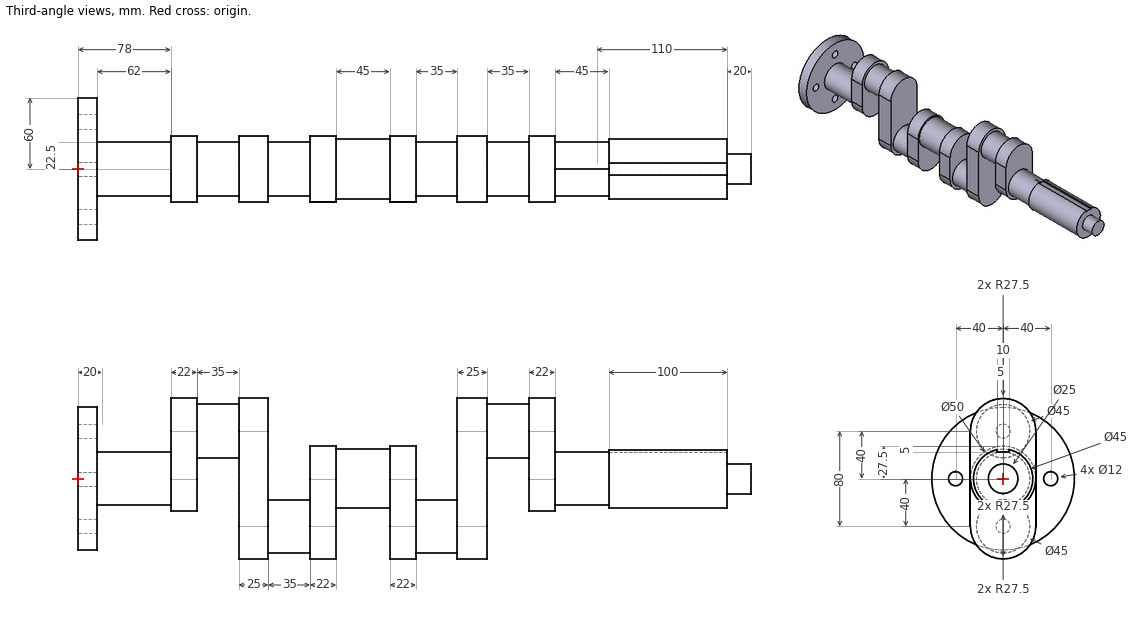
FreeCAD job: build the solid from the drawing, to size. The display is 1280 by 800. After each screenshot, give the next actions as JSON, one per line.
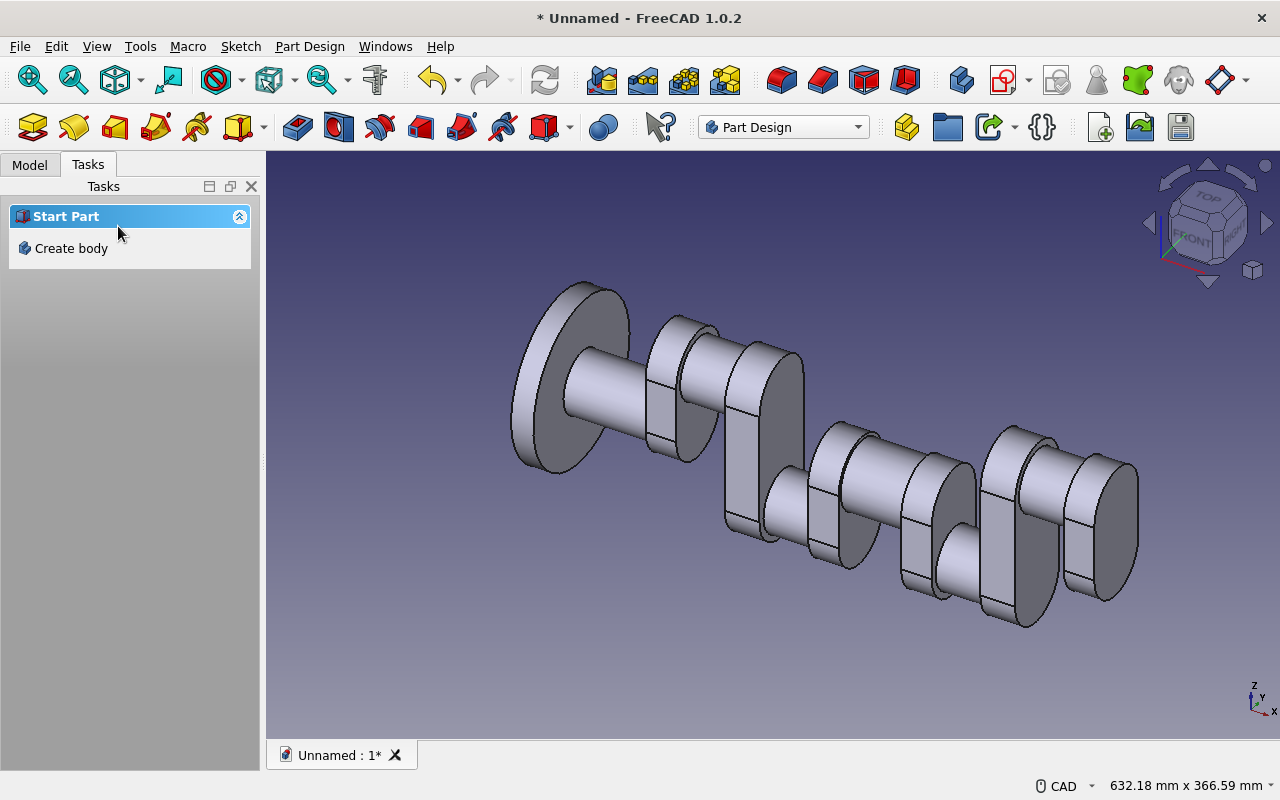
{"action": "left_click", "coordinate": [30, 164]}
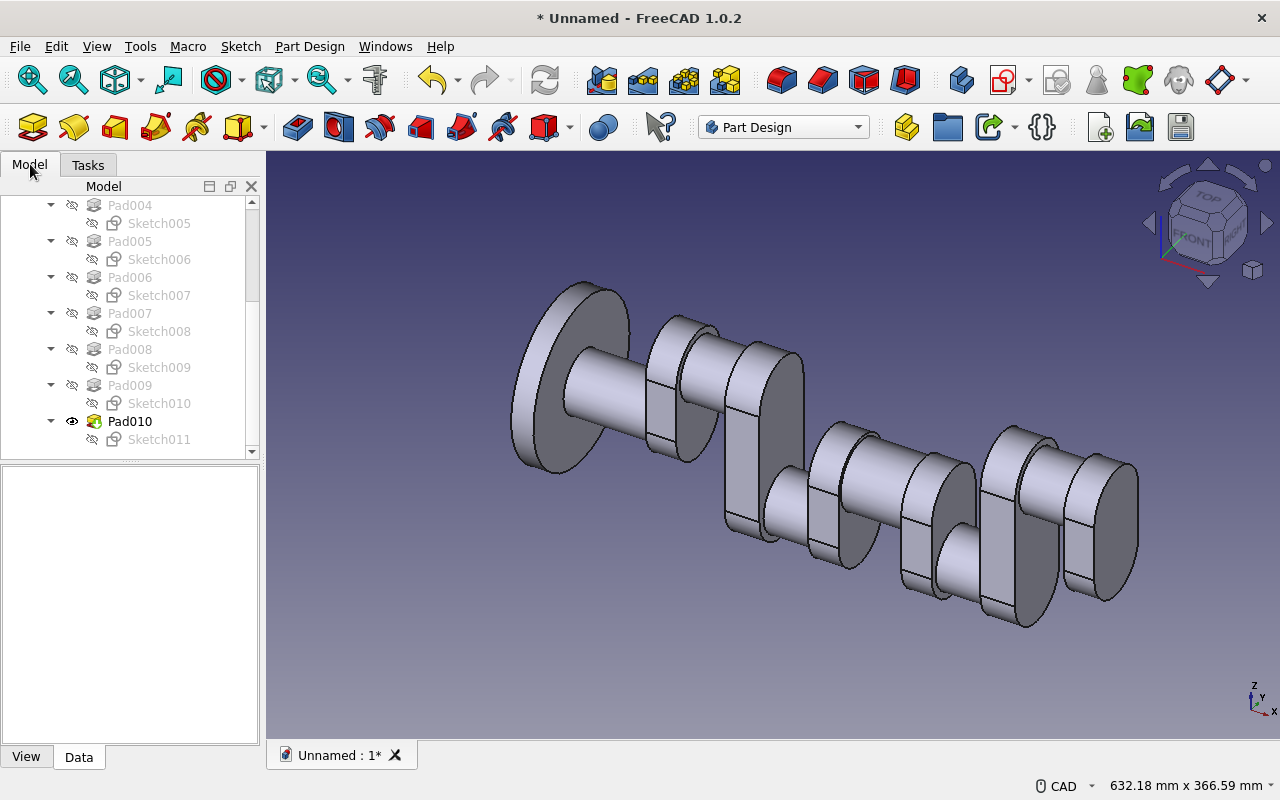
{"action": "scroll", "coordinate": [141, 327], "scroll_direction": "down", "scroll_amount": 3}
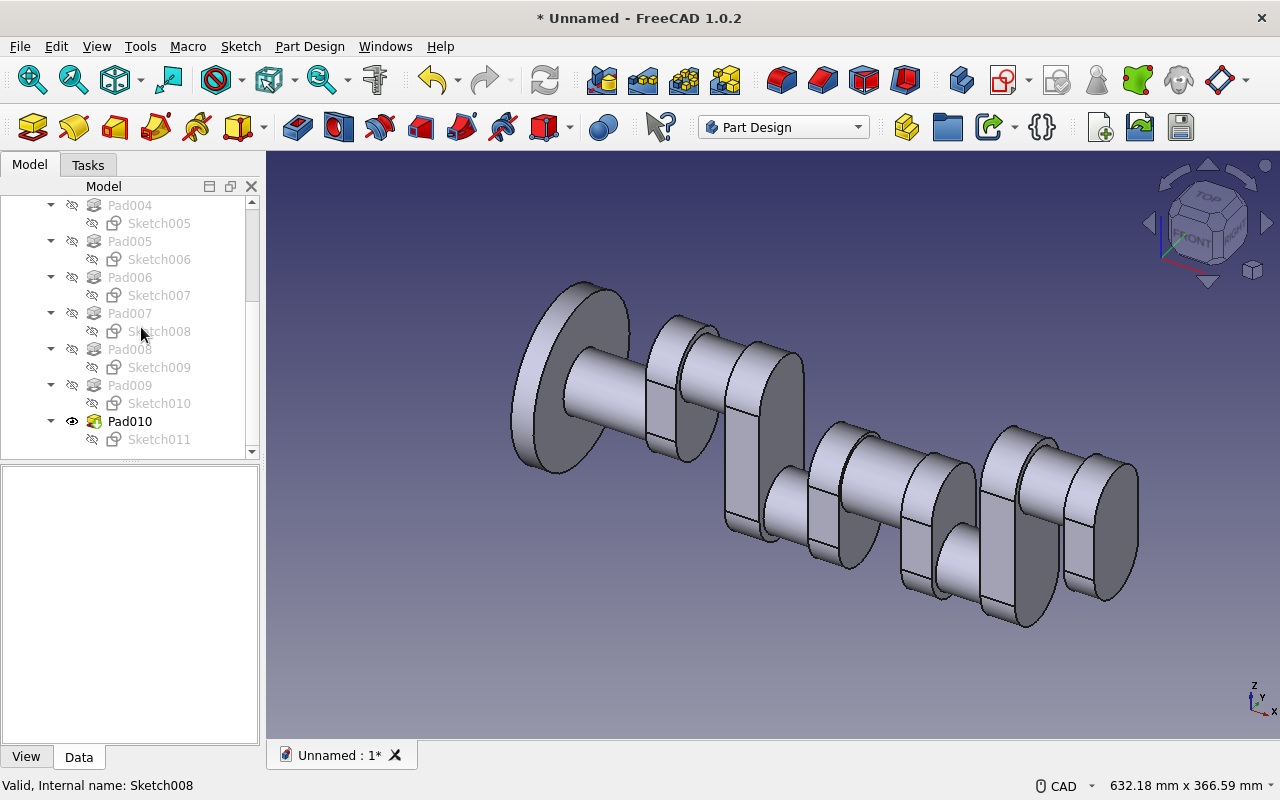
{"action": "scroll", "coordinate": [141, 327], "scroll_direction": "up", "scroll_amount": 15}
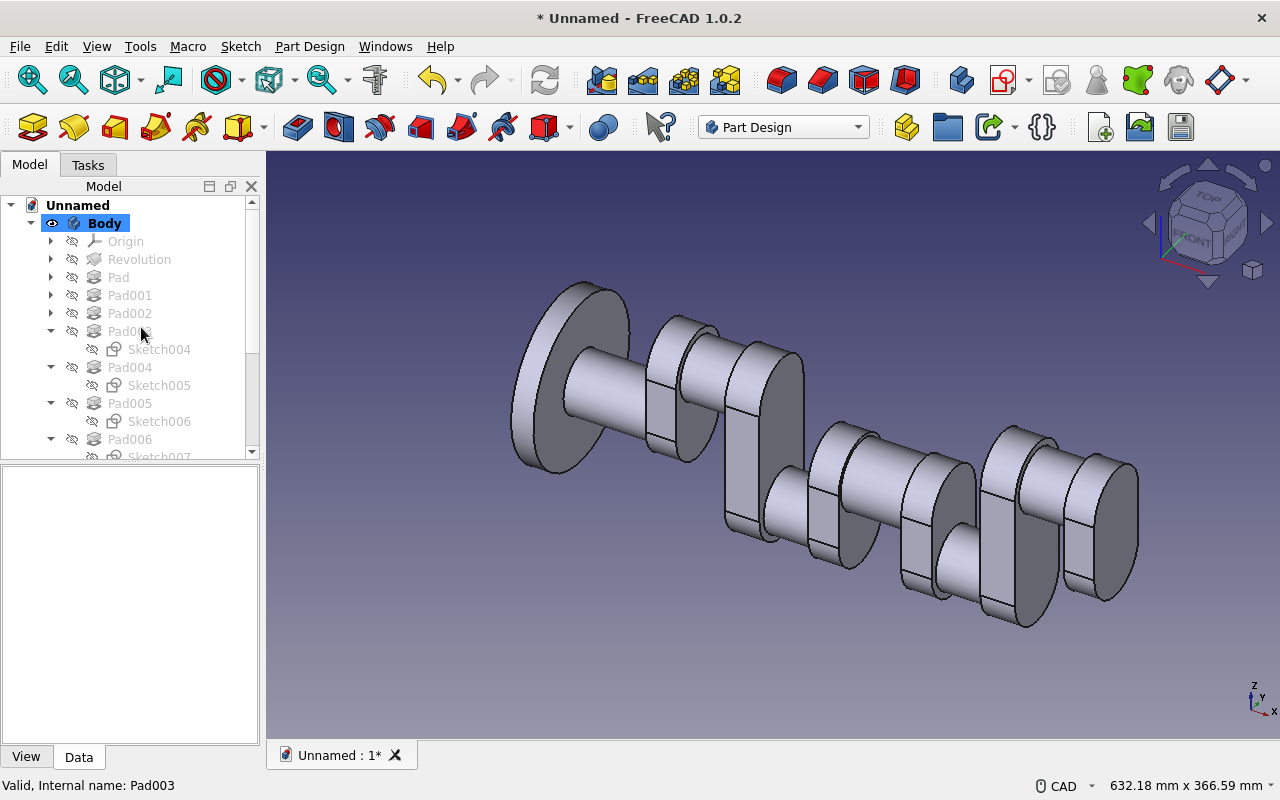
{"action": "left_click", "coordinate": [51, 241]}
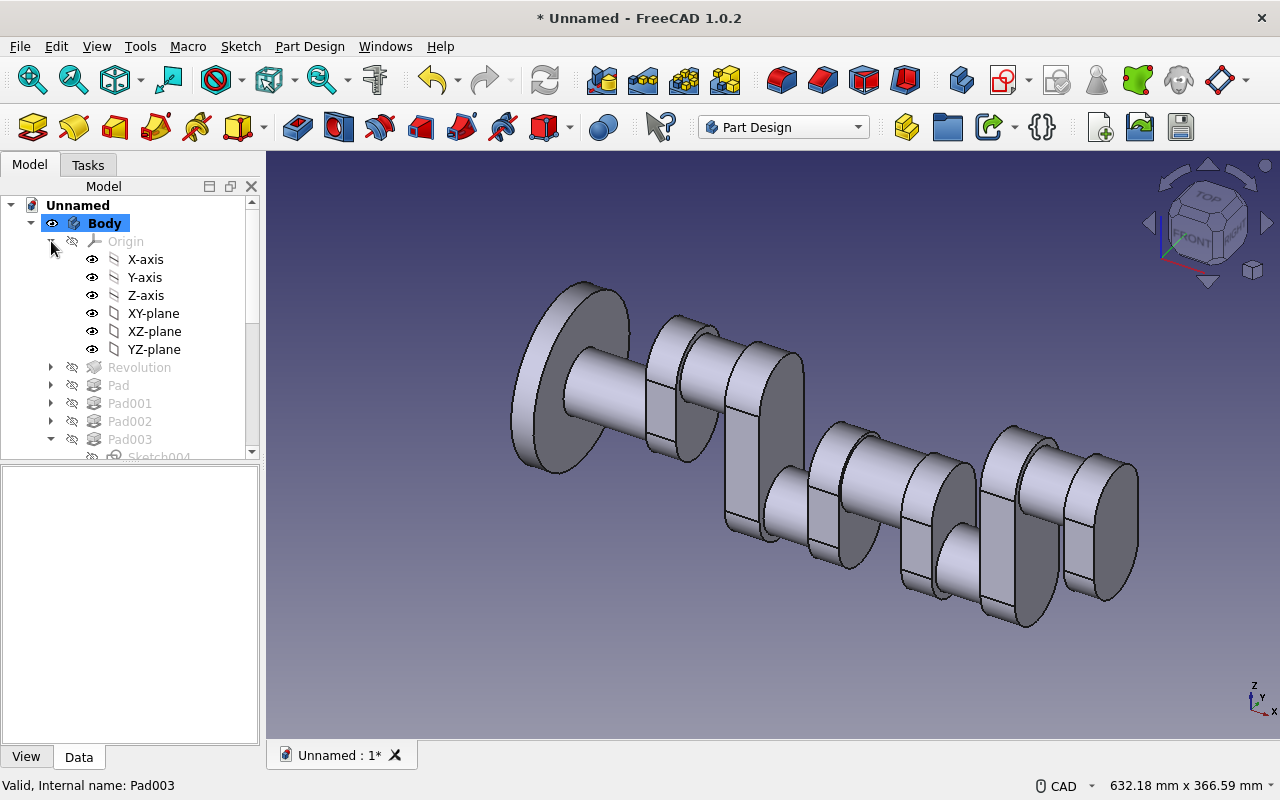
{"action": "left_click", "coordinate": [137, 349]}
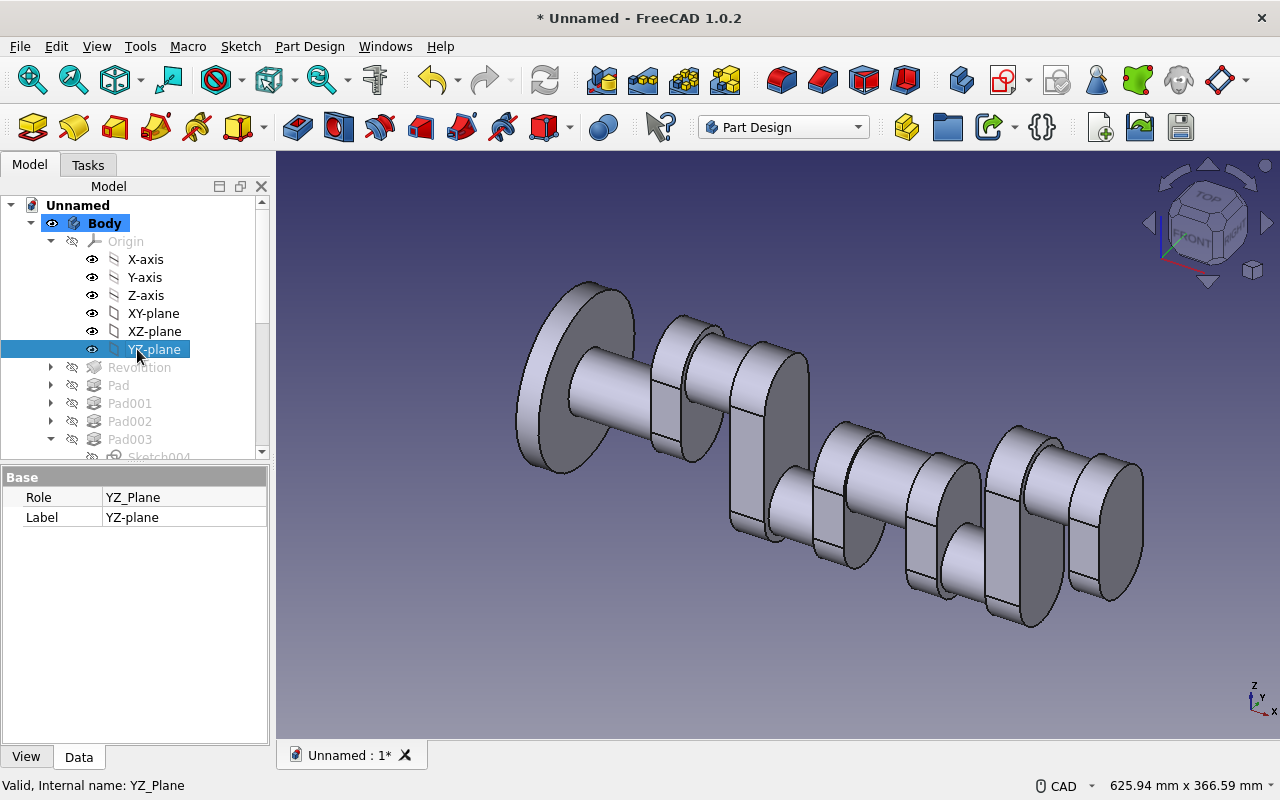
{"action": "left_click", "coordinate": [1220, 80]}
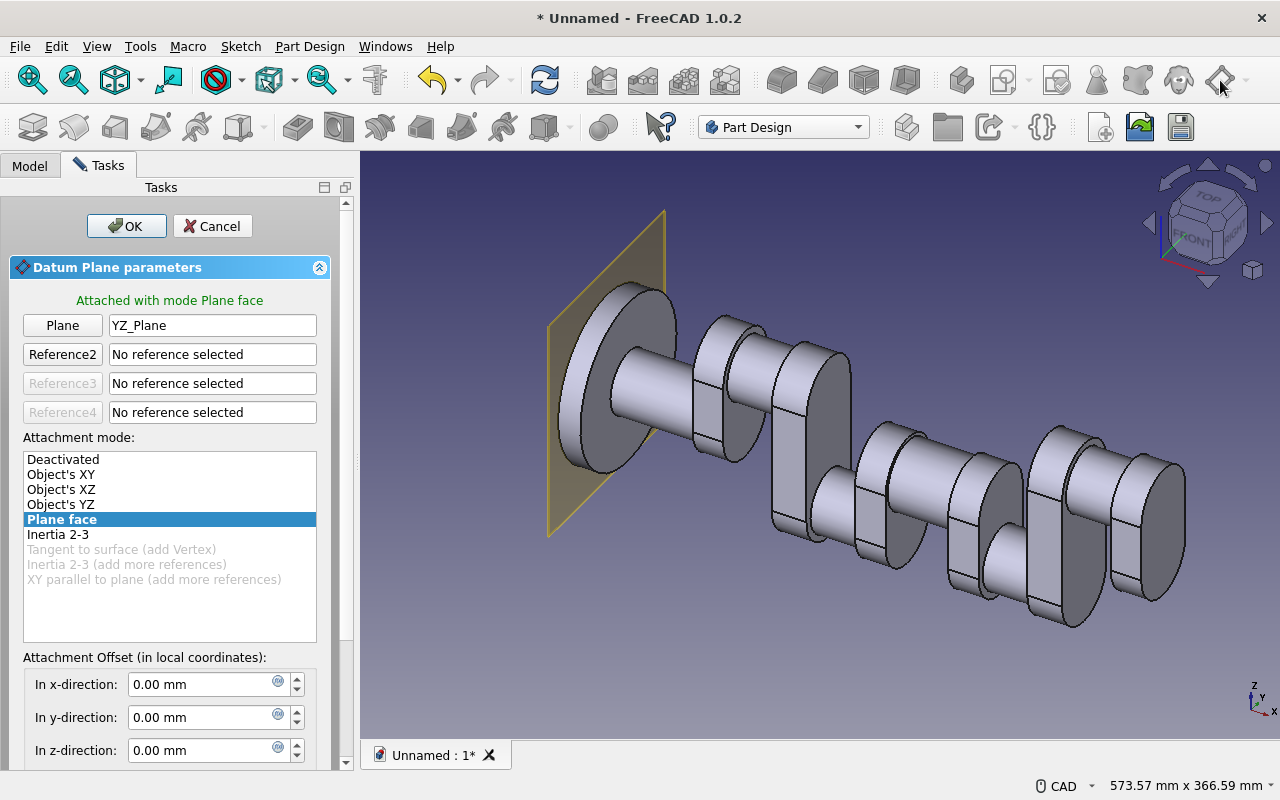
{"action": "triple_click", "coordinate": [210, 750]}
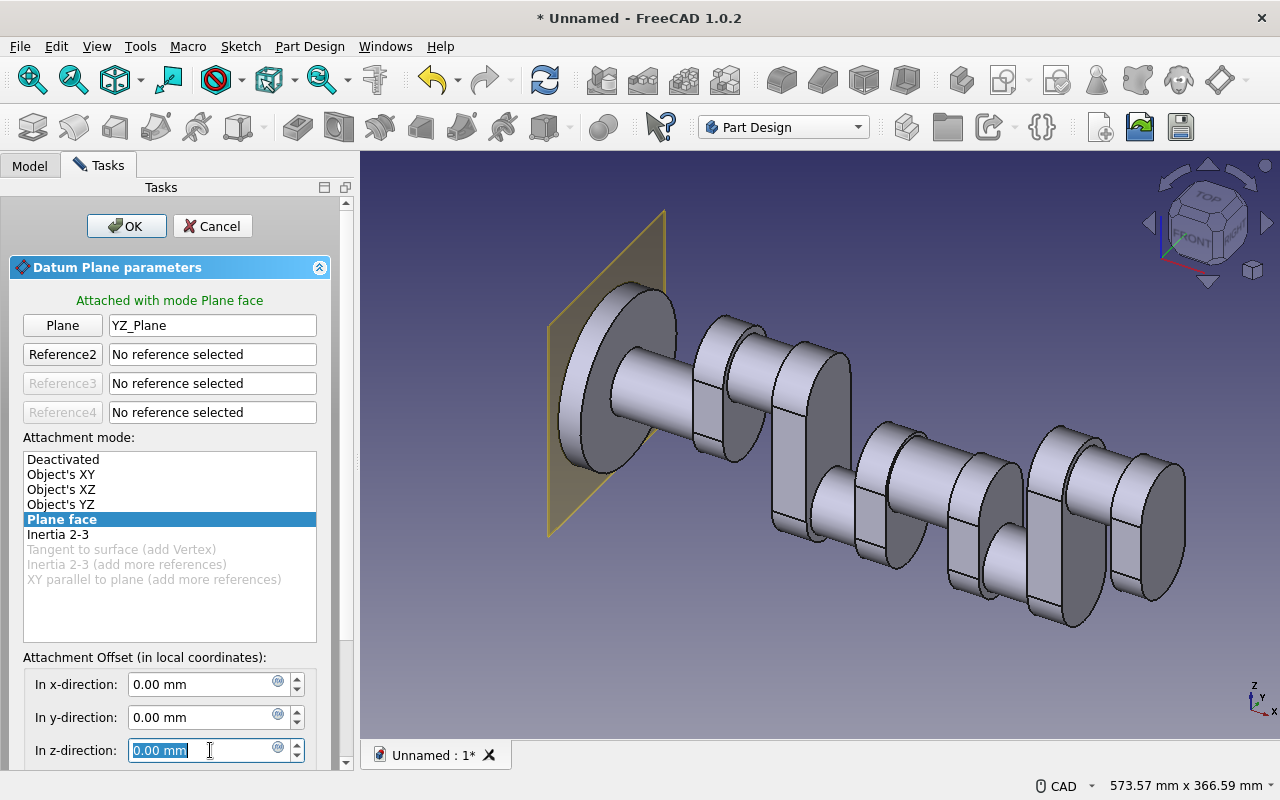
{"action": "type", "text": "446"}
{"action": "key", "text": "Tab"}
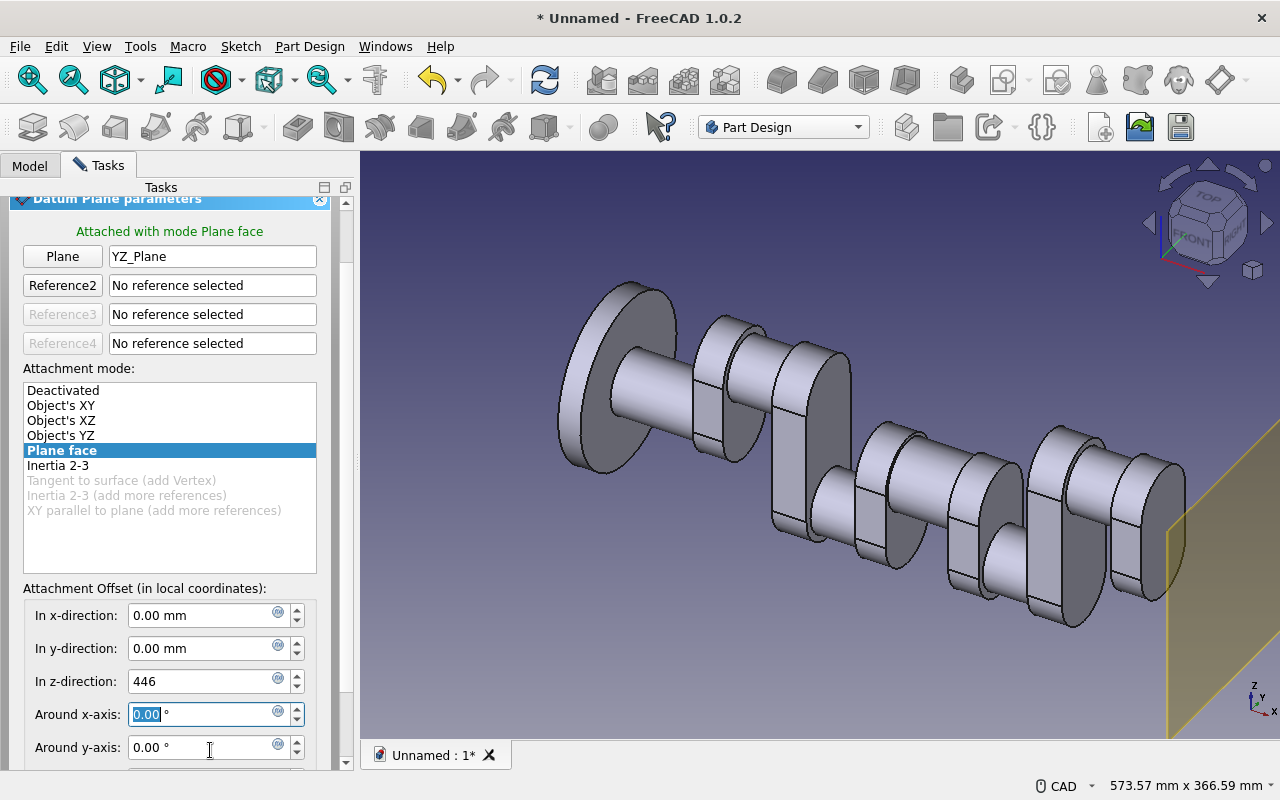
{"action": "scroll", "coordinate": [346, 484], "scroll_direction": "up", "scroll_amount": 2}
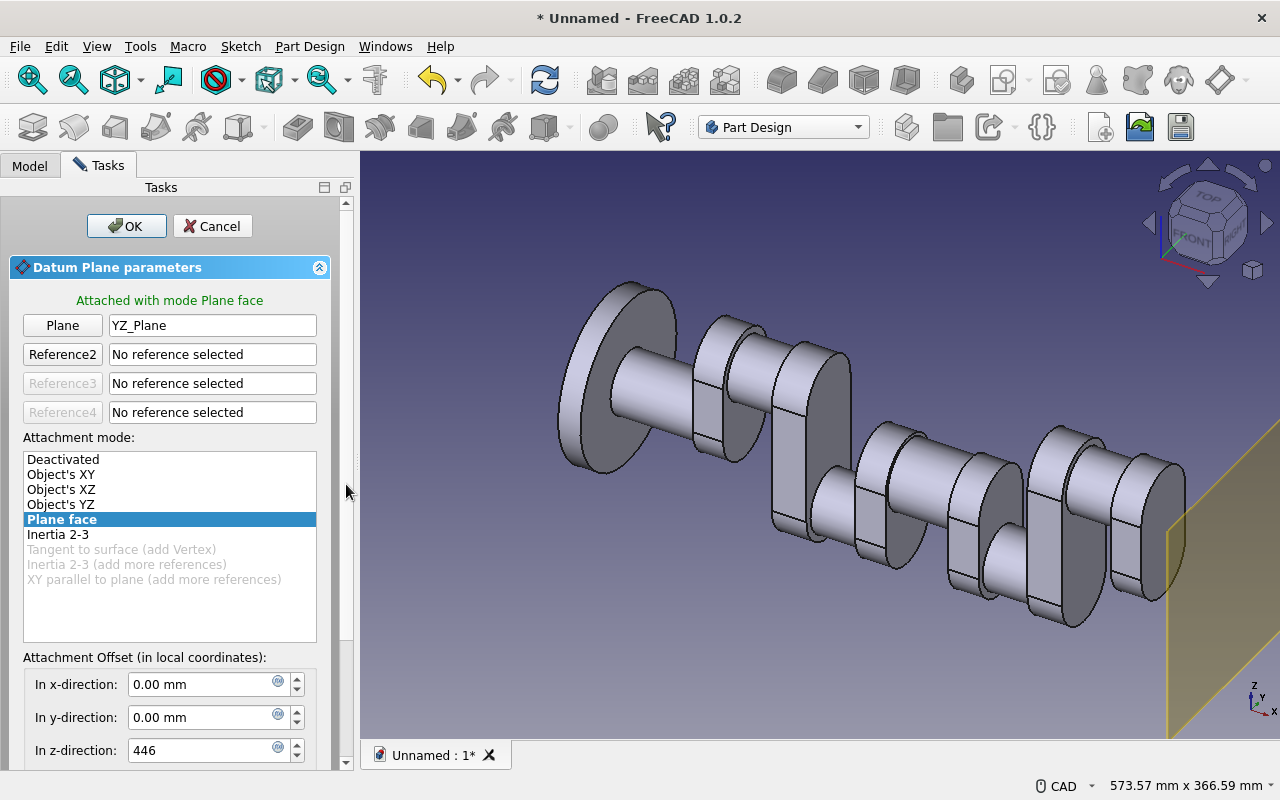
{"action": "left_click", "coordinate": [127, 226]}